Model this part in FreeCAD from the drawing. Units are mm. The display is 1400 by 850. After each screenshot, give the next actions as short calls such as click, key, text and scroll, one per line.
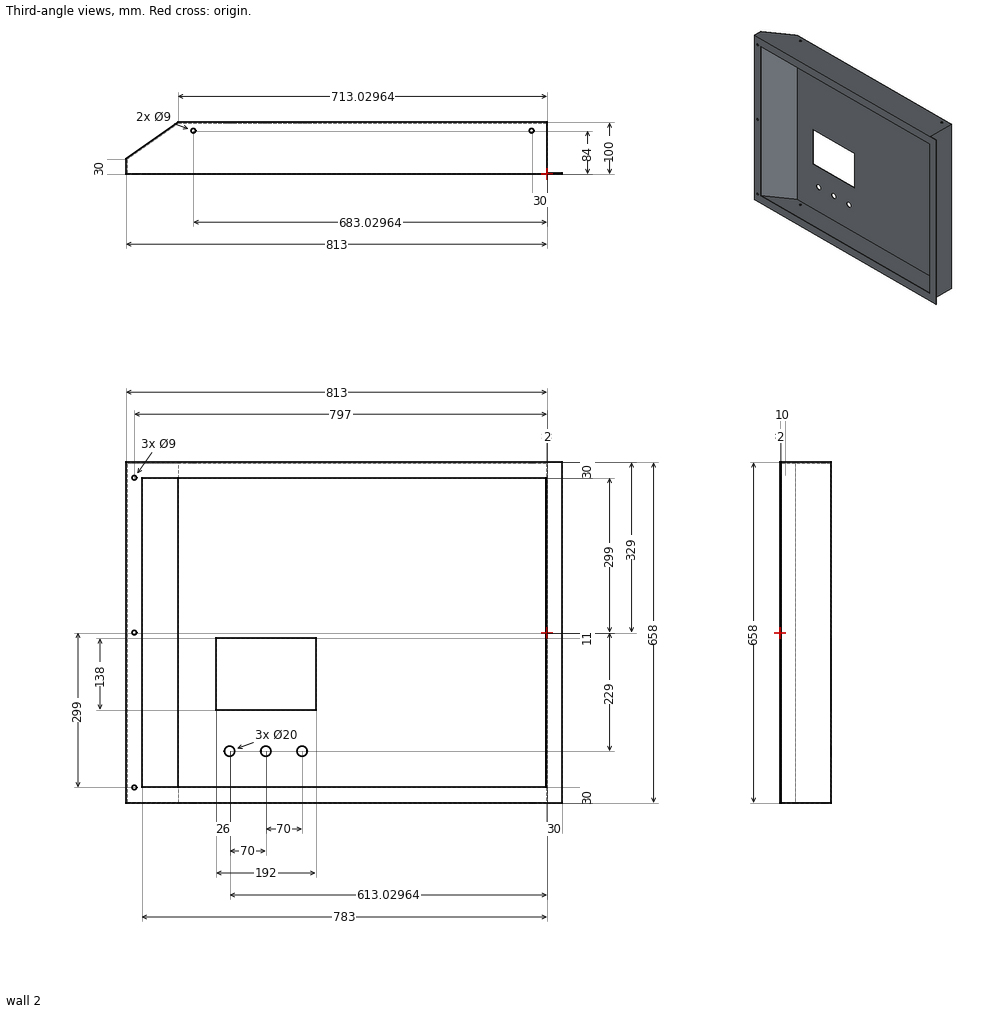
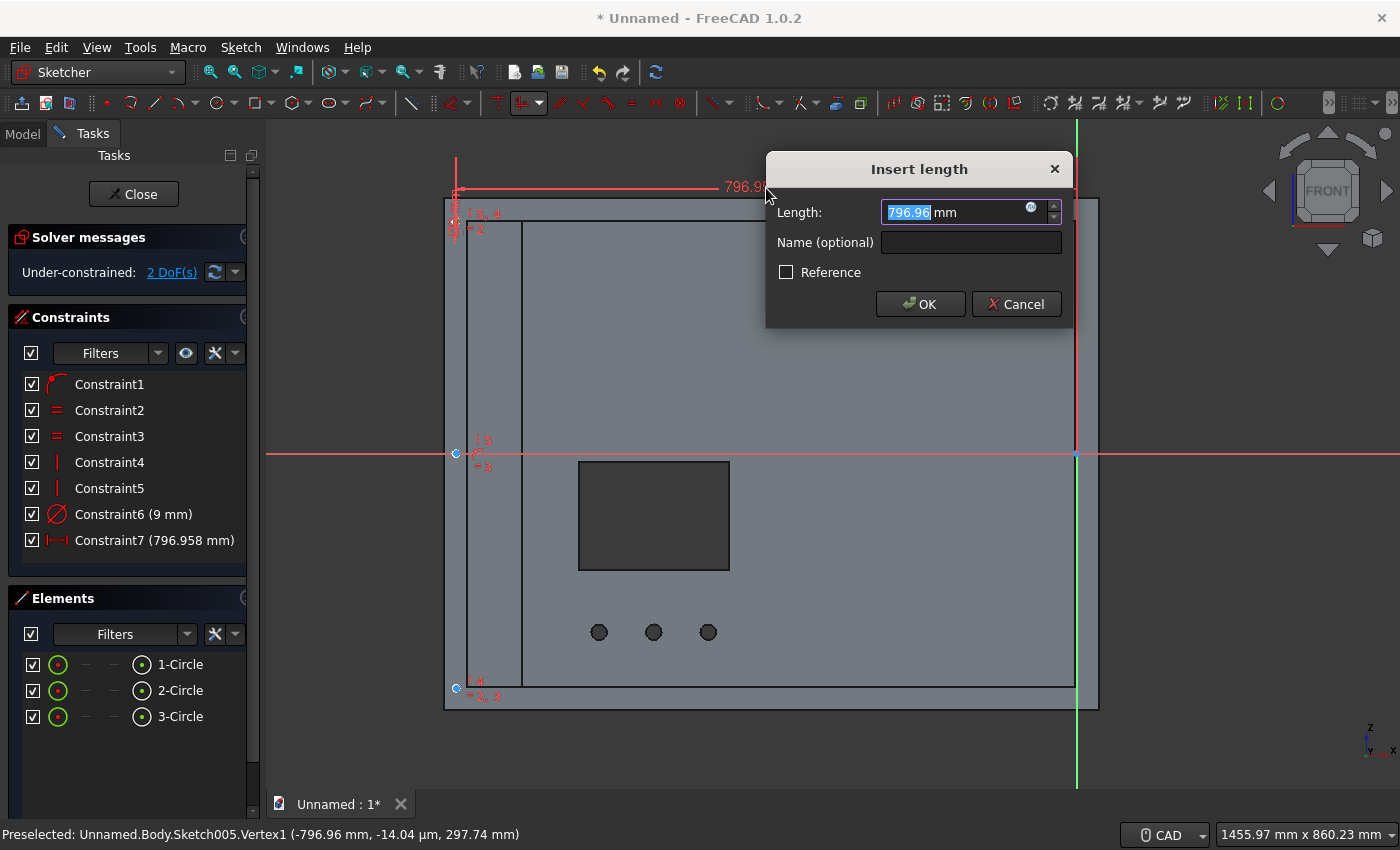
text(797)
key(Return)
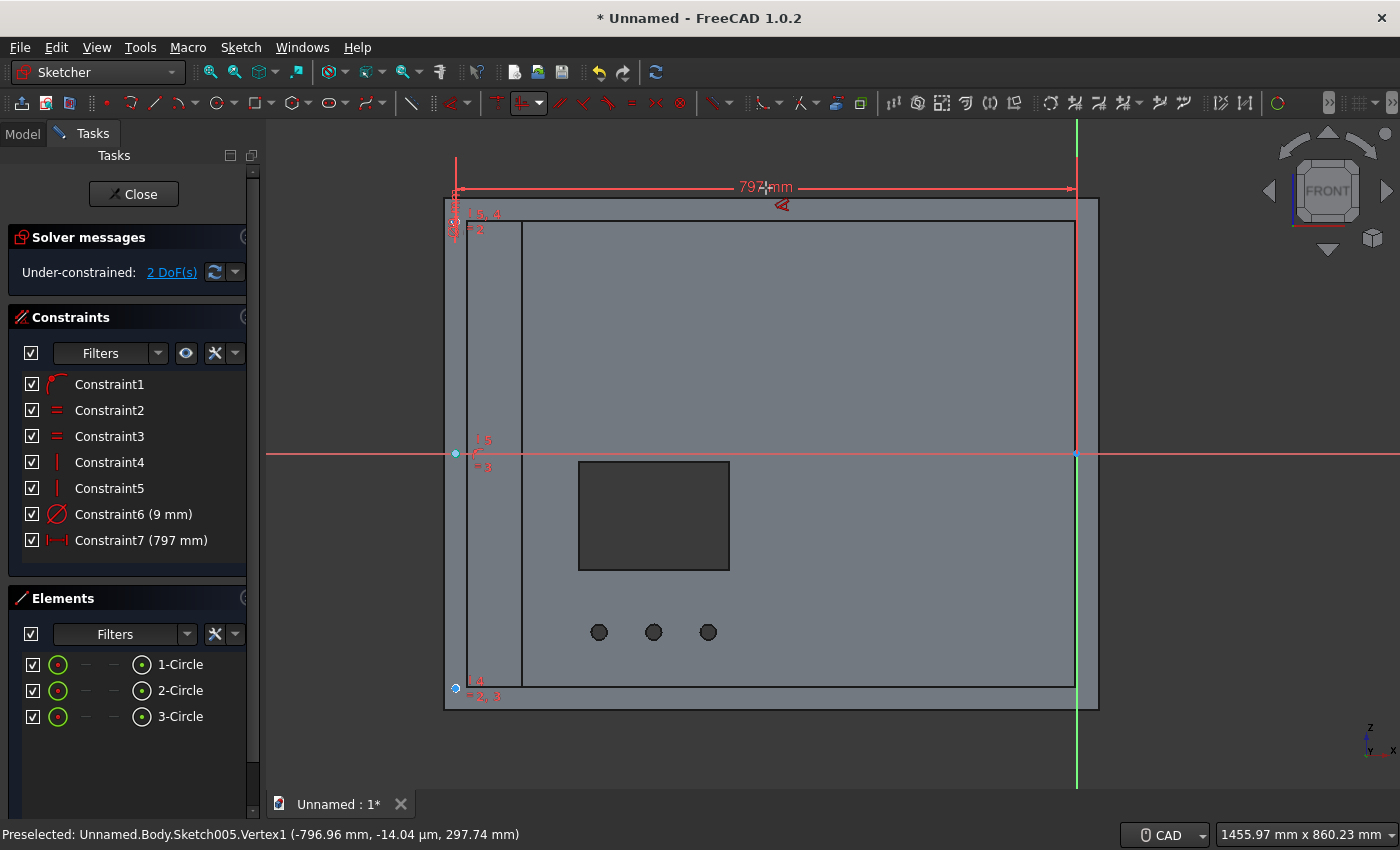
click(456, 222)
click(1111, 338)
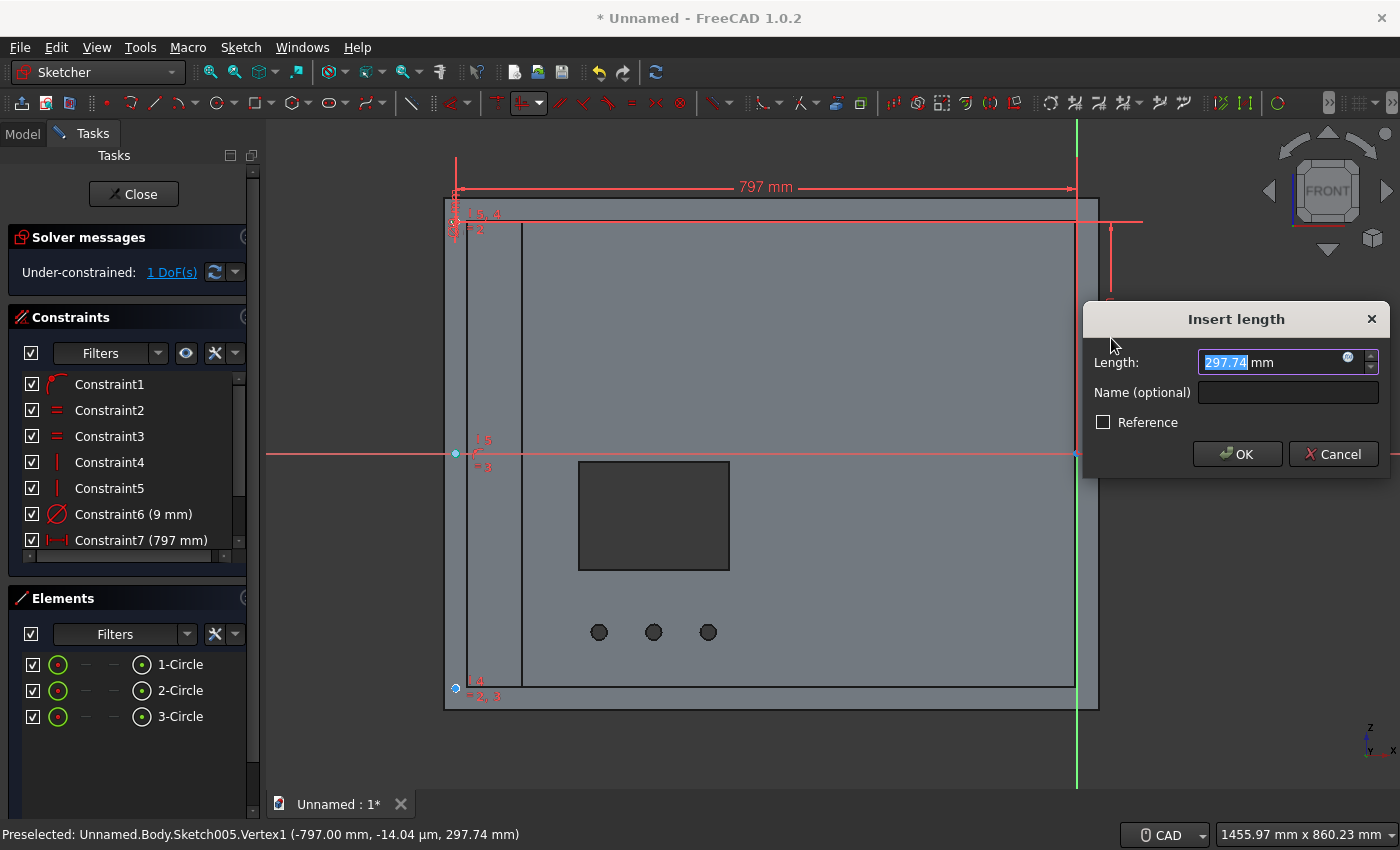
text(299)
key(Return)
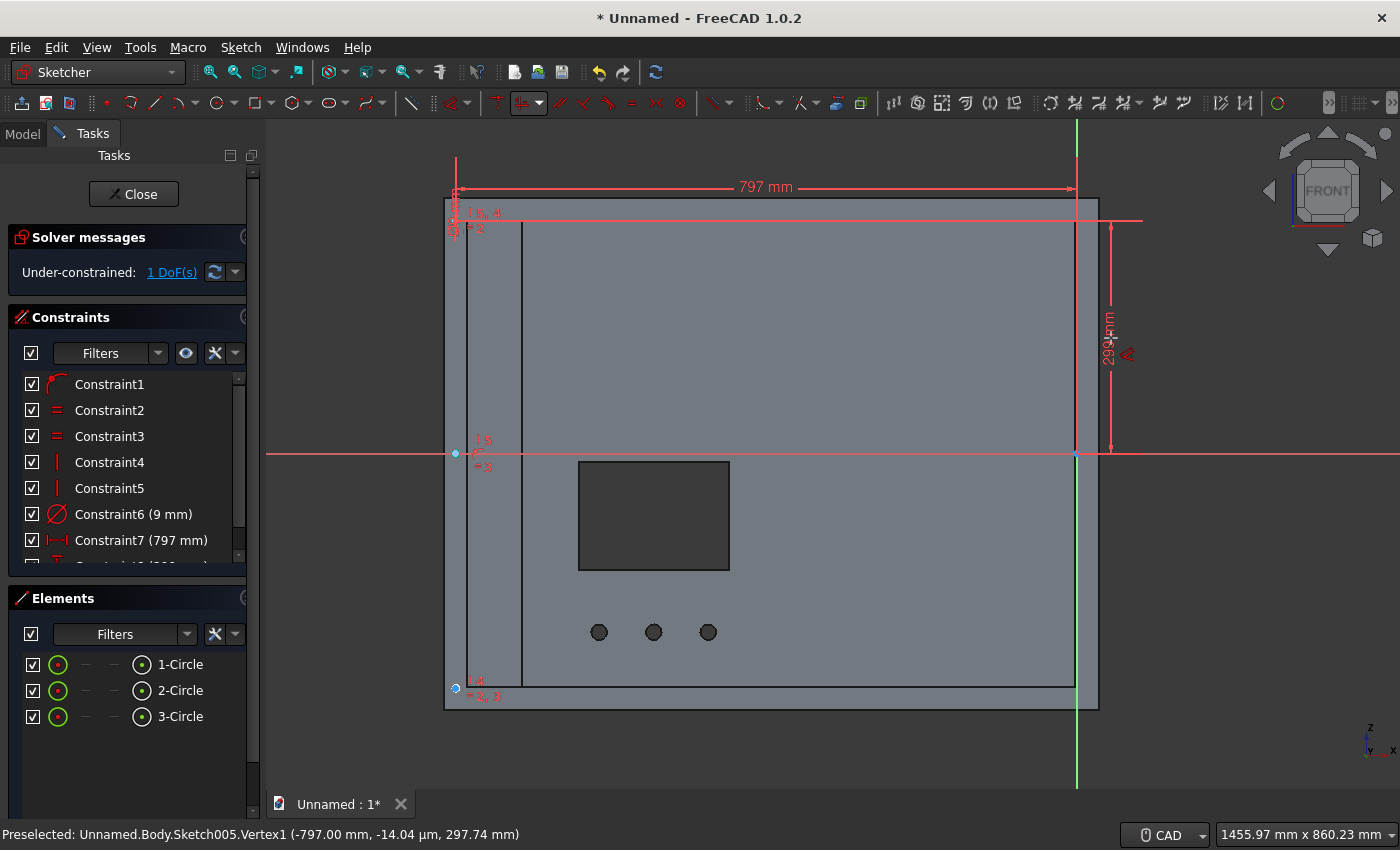
click(456, 688)
click(1111, 571)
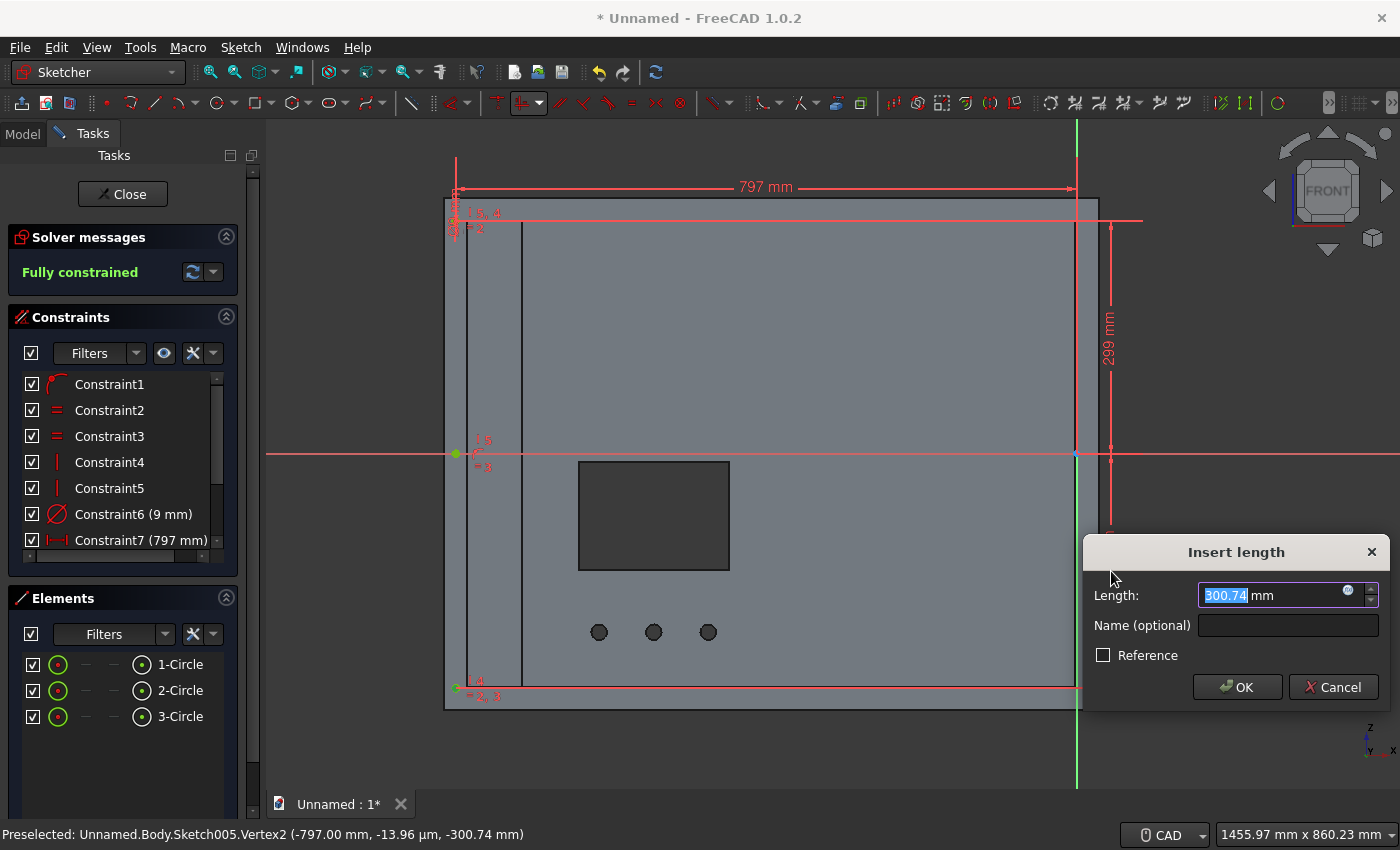
text(299)
key(Return)
key(Escape)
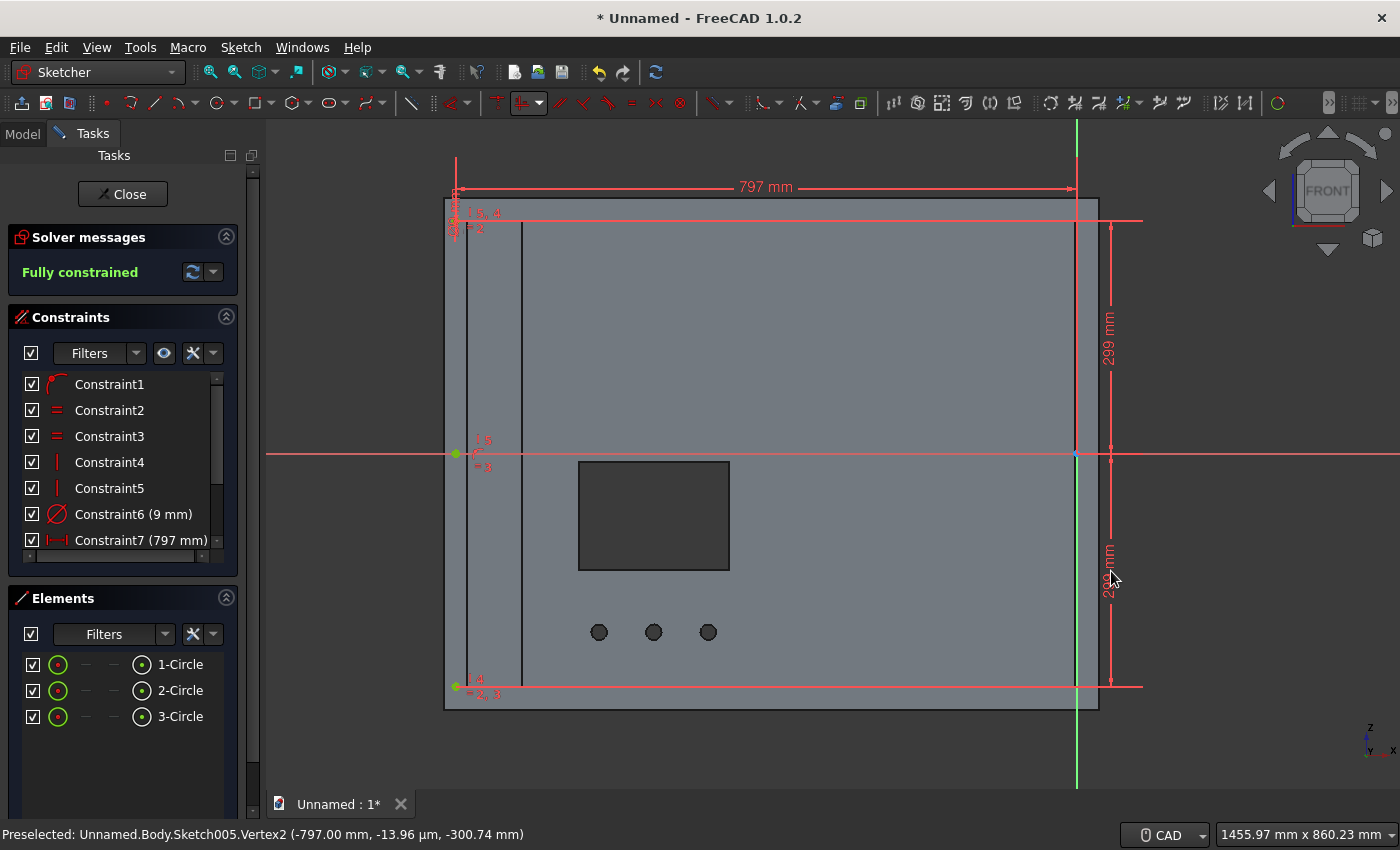
click(123, 194)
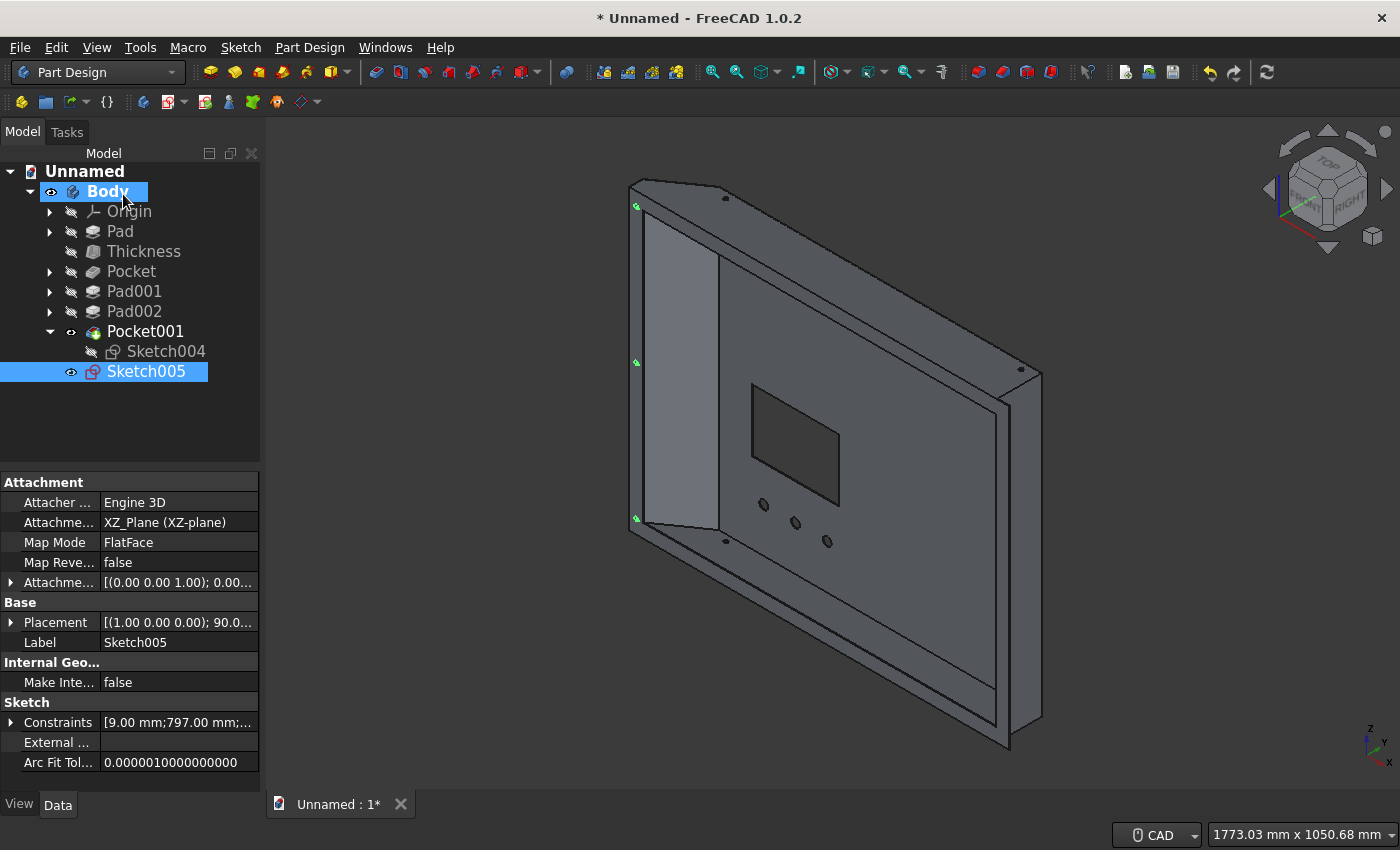
click(378, 72)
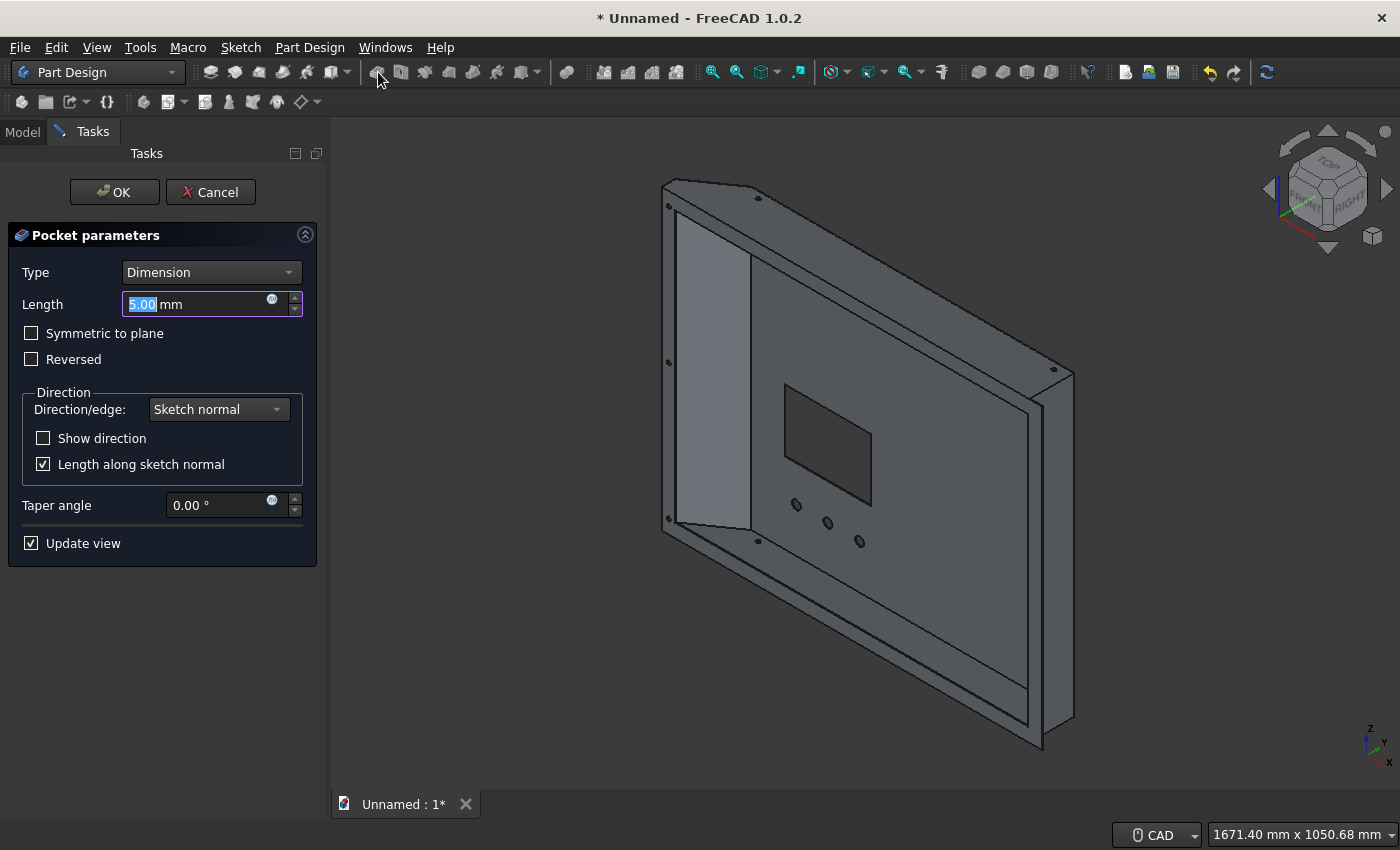
text(10)
key(Tab)